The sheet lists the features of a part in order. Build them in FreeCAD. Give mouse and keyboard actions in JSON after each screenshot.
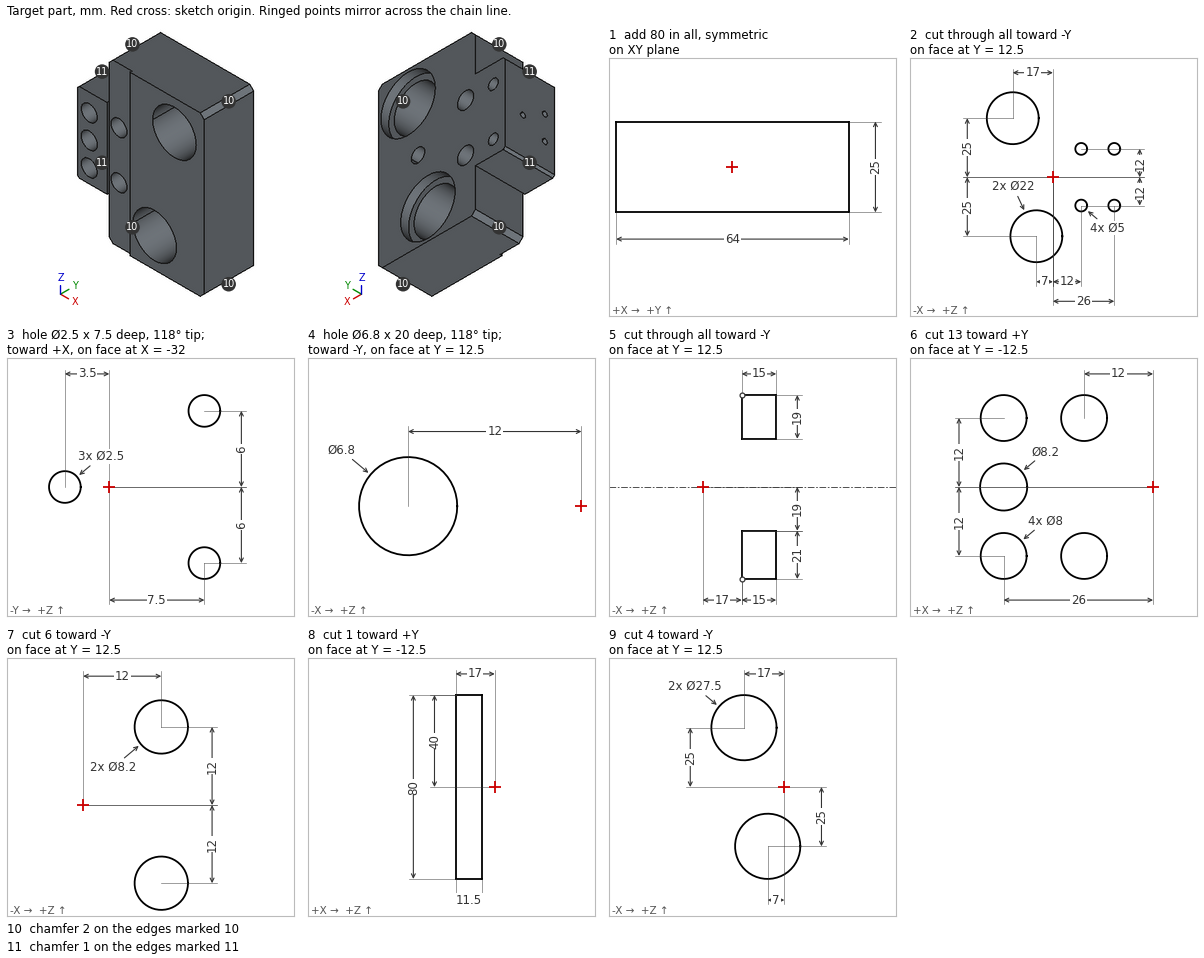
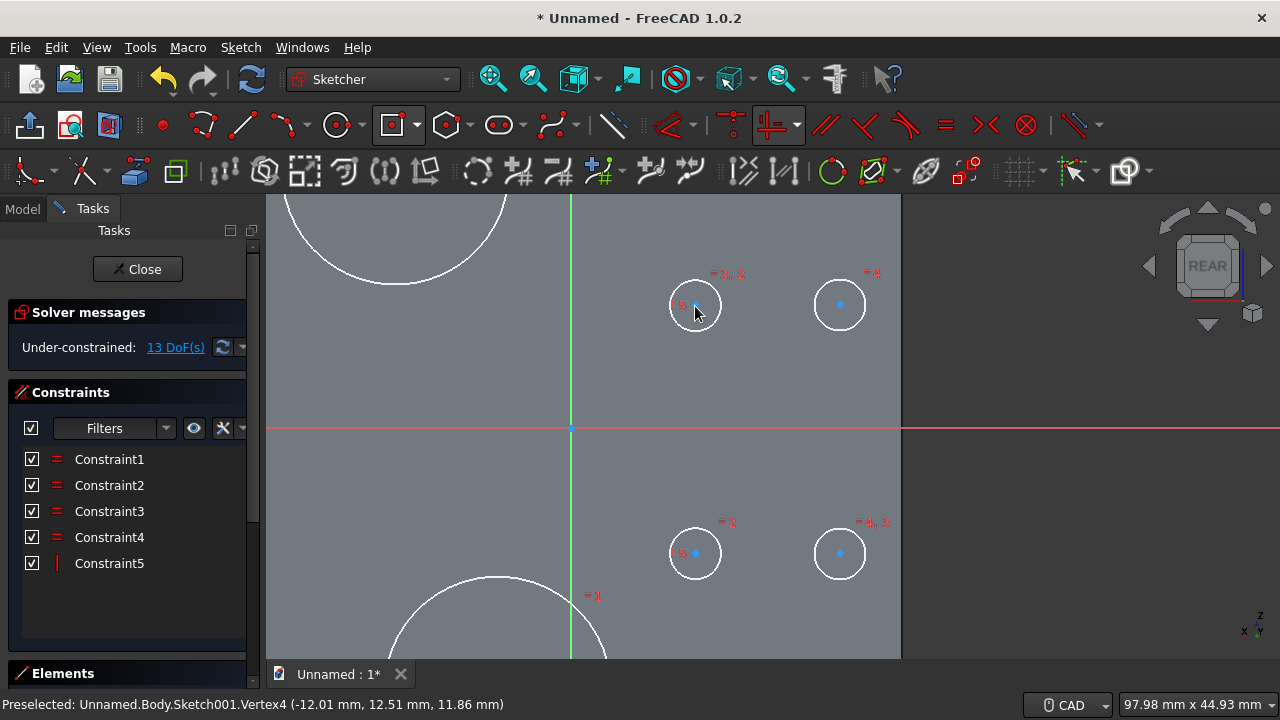
{"action": "left_click", "coordinate": [695, 554]}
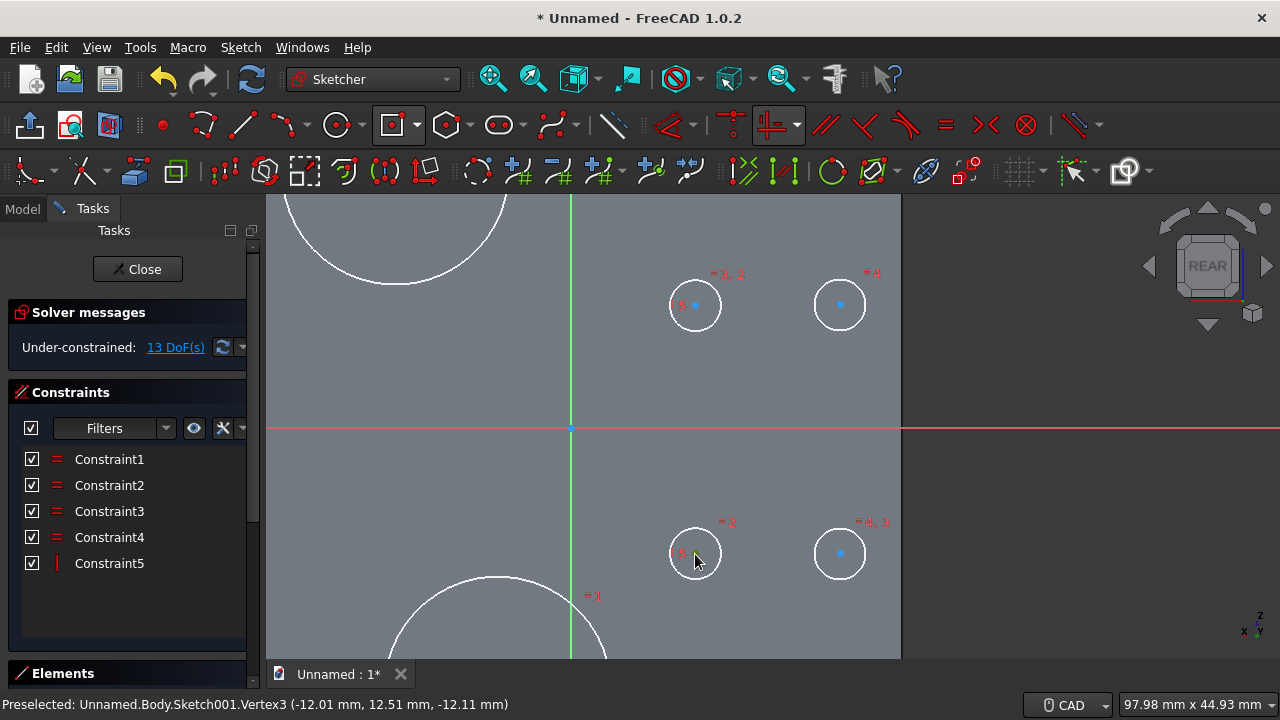
{"action": "left_click", "coordinate": [840, 554]}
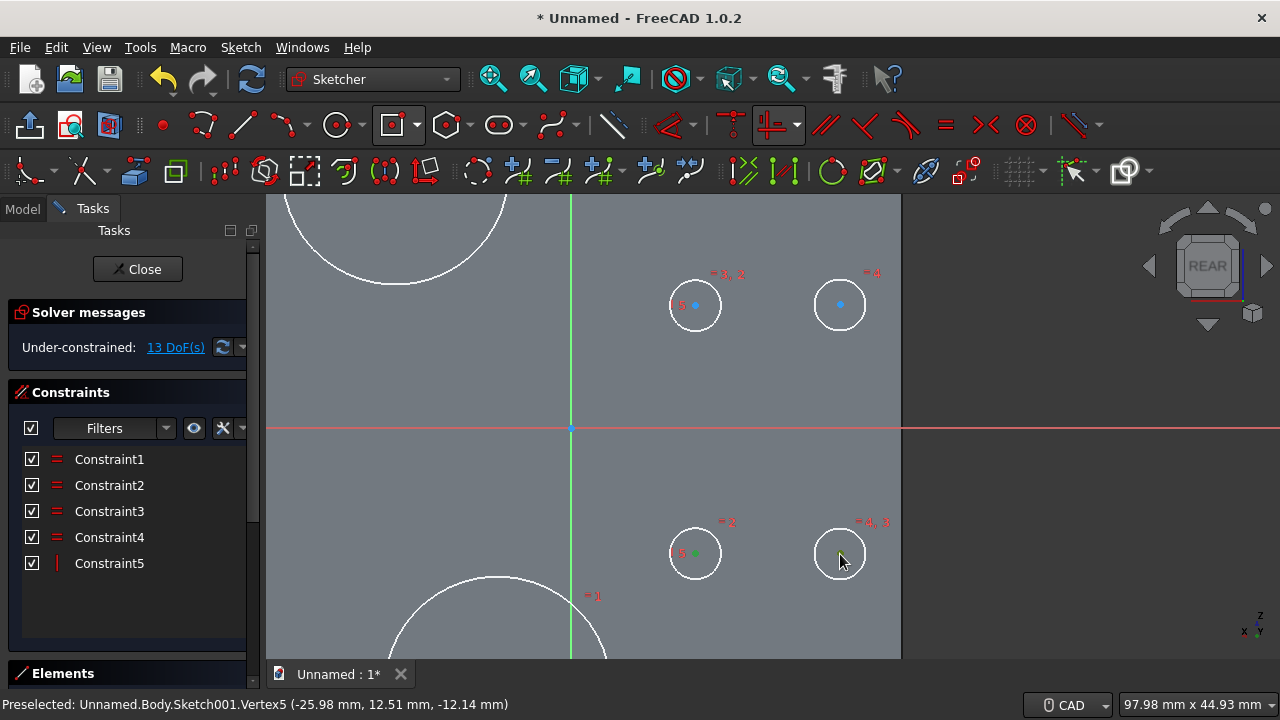
{"action": "key", "text": "h"}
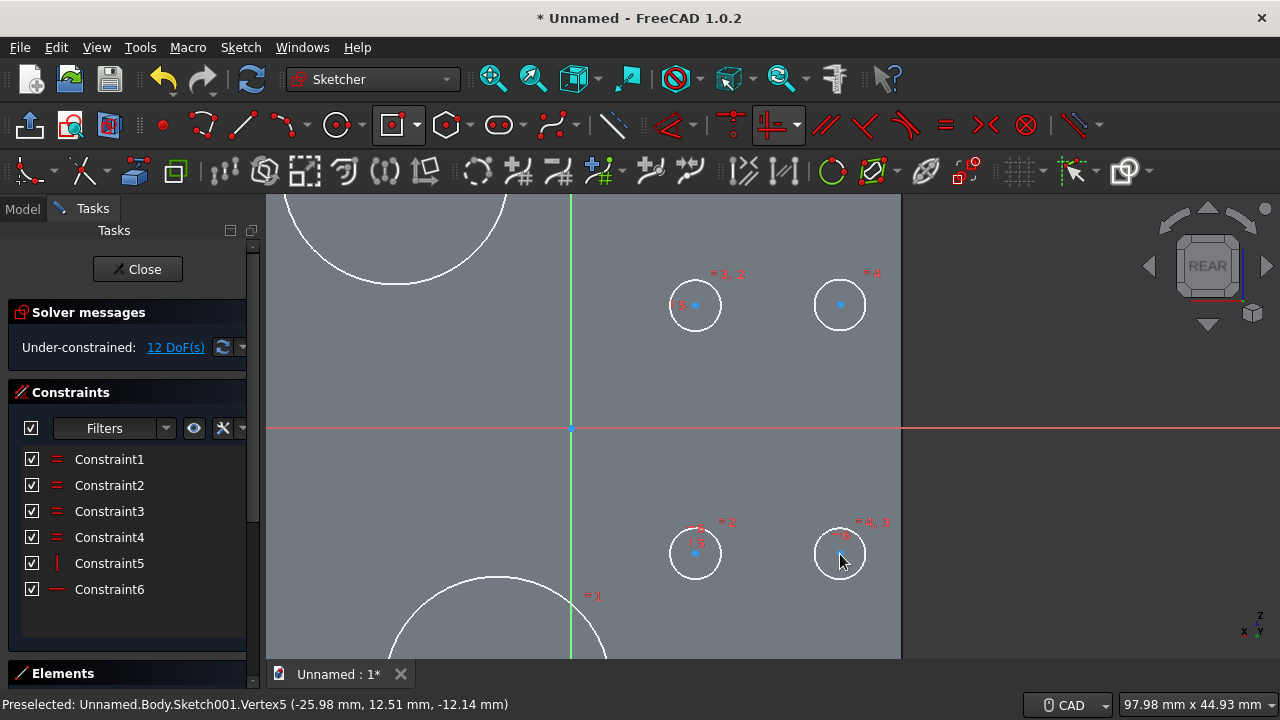
{"action": "left_click", "coordinate": [840, 554]}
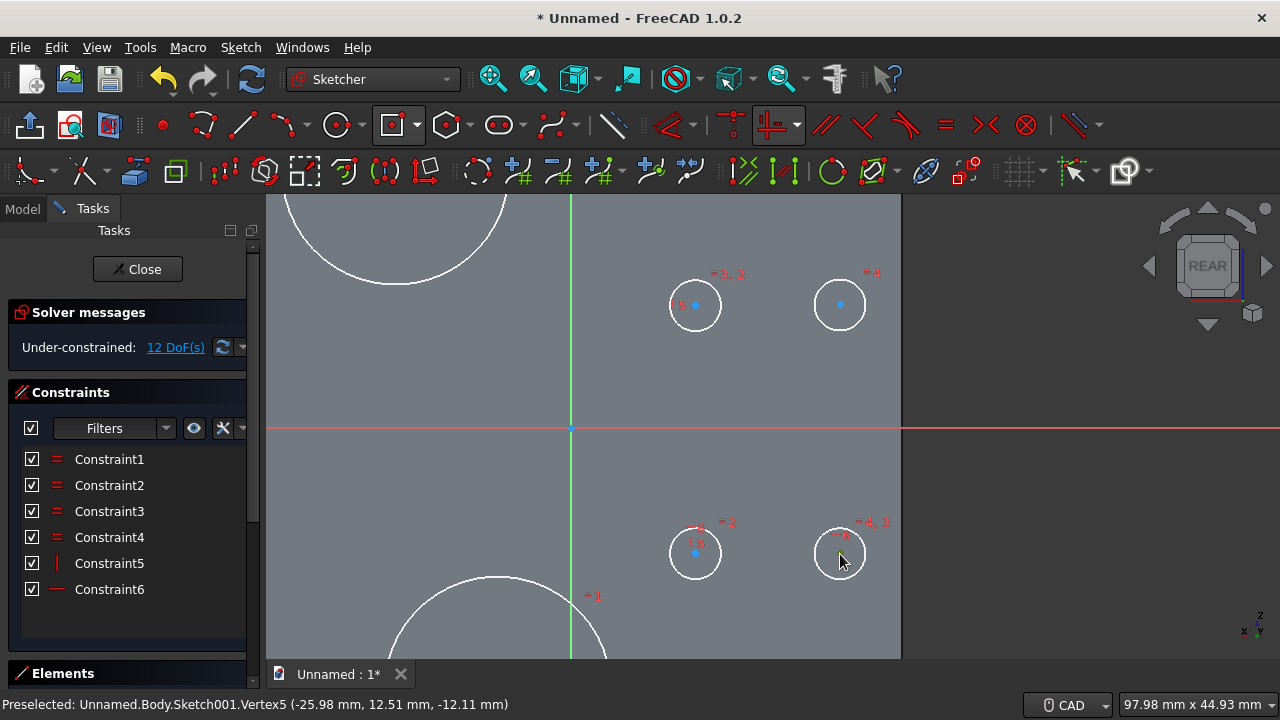
{"action": "left_click", "coordinate": [840, 305]}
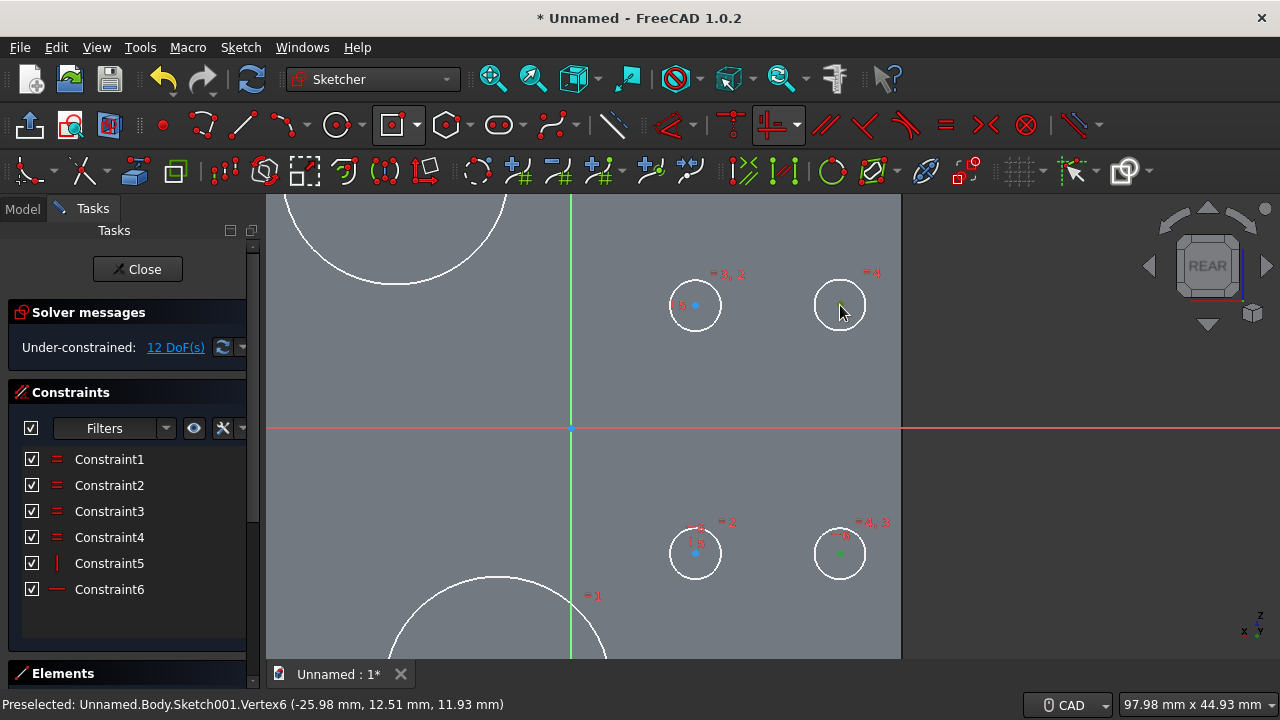
{"action": "left_click", "coordinate": [800, 126]}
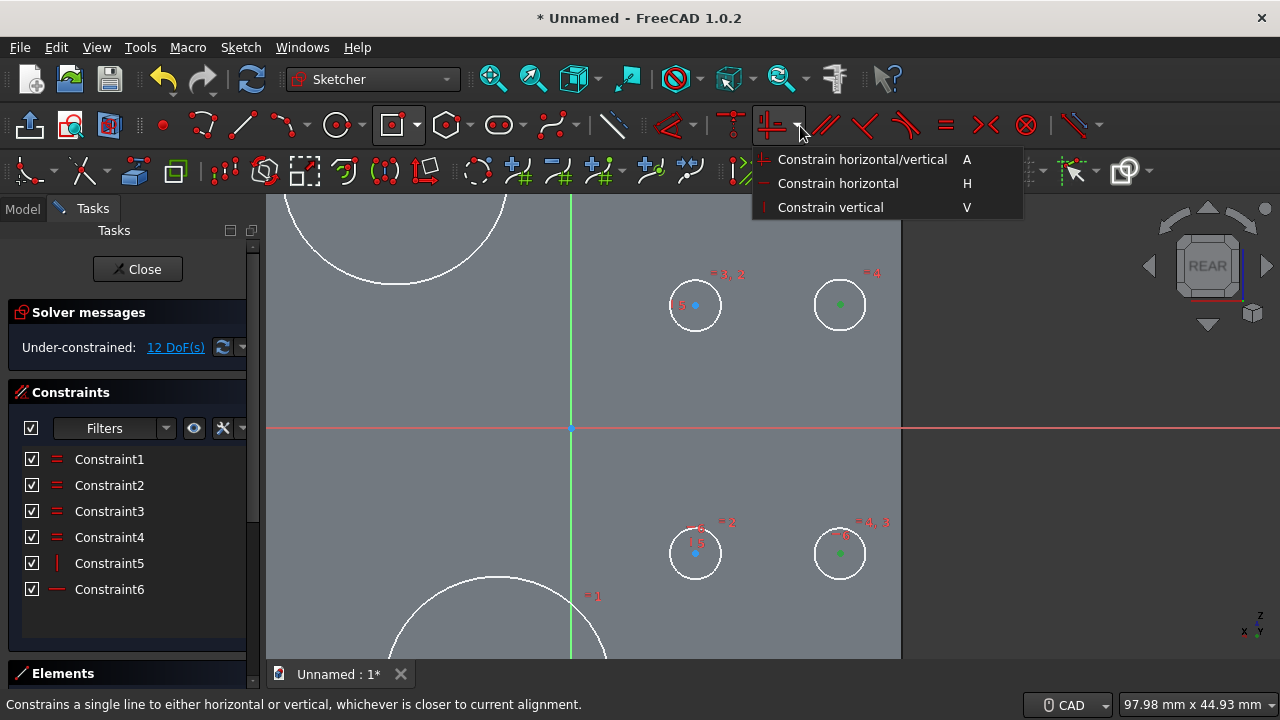
{"action": "left_click", "coordinate": [888, 207]}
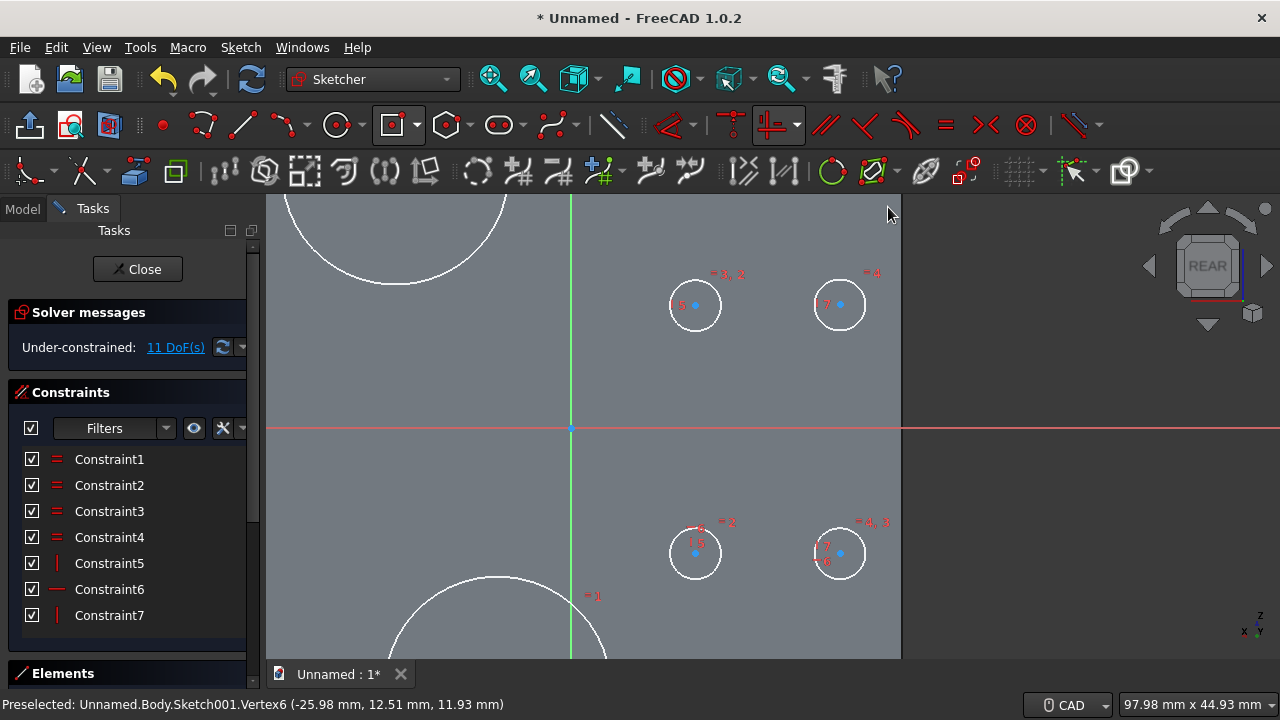
{"action": "left_click", "coordinate": [695, 306]}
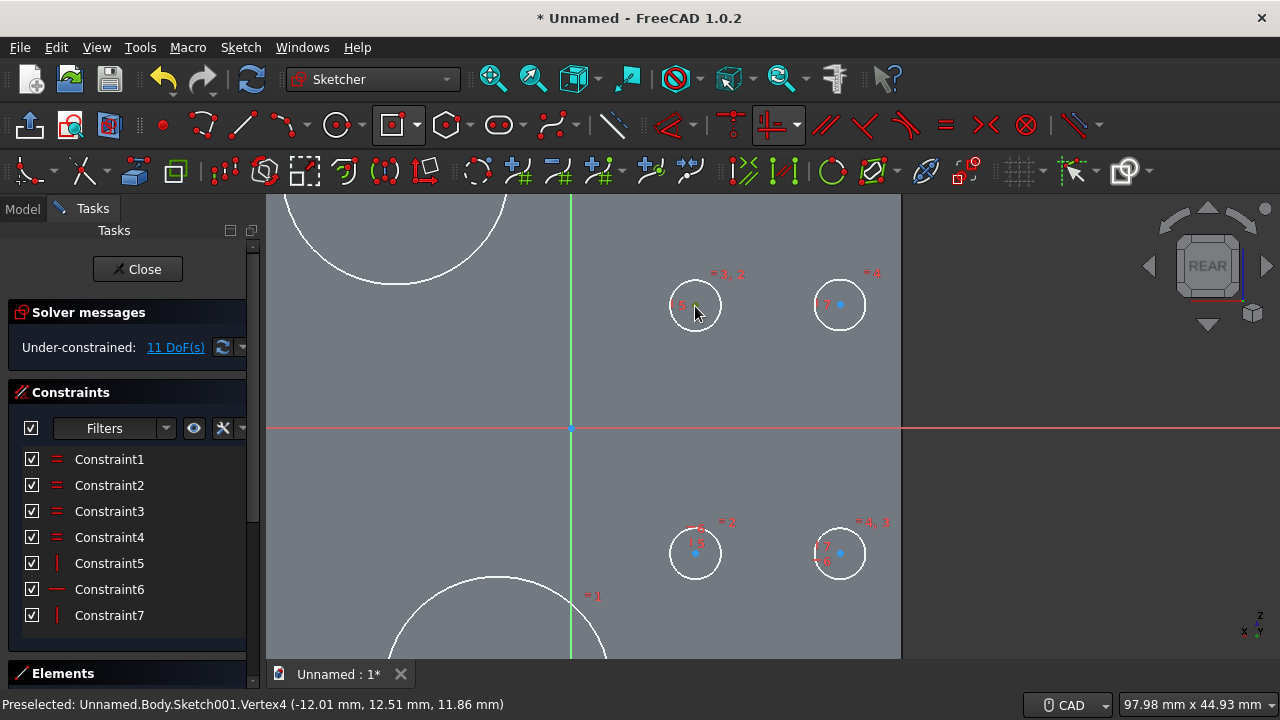
{"action": "left_click", "coordinate": [840, 305]}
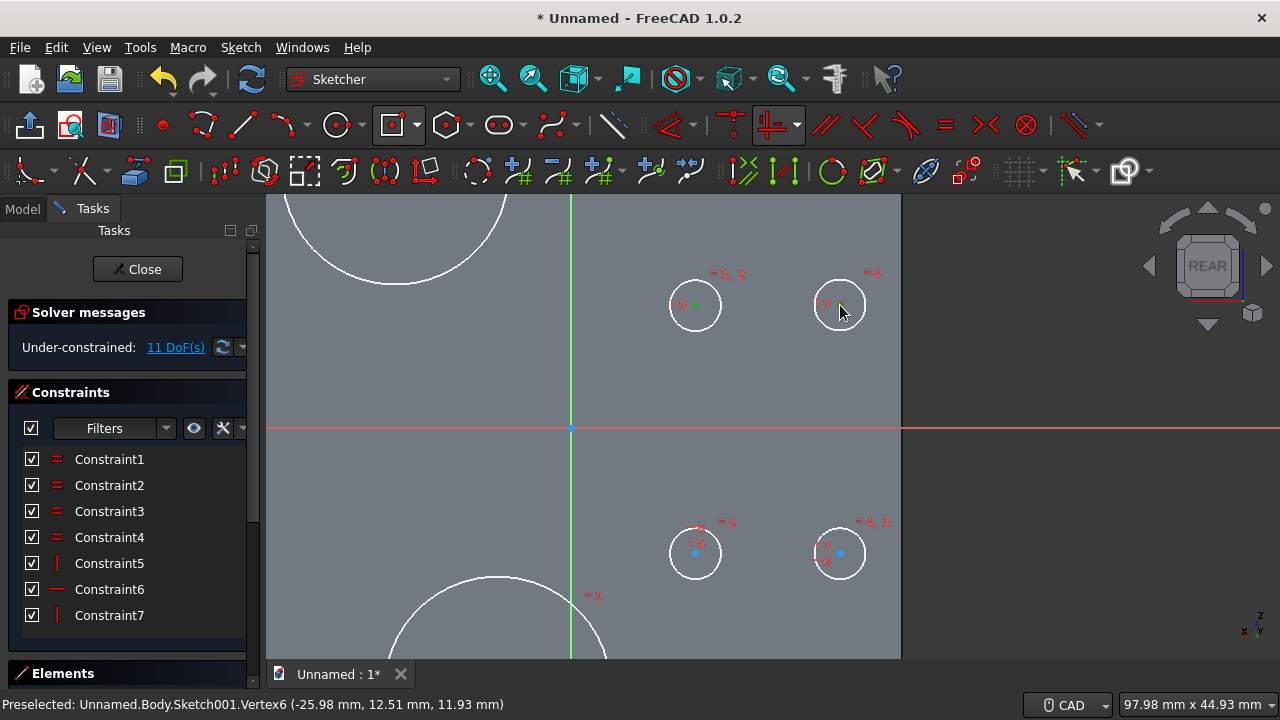
{"action": "left_click", "coordinate": [800, 126]}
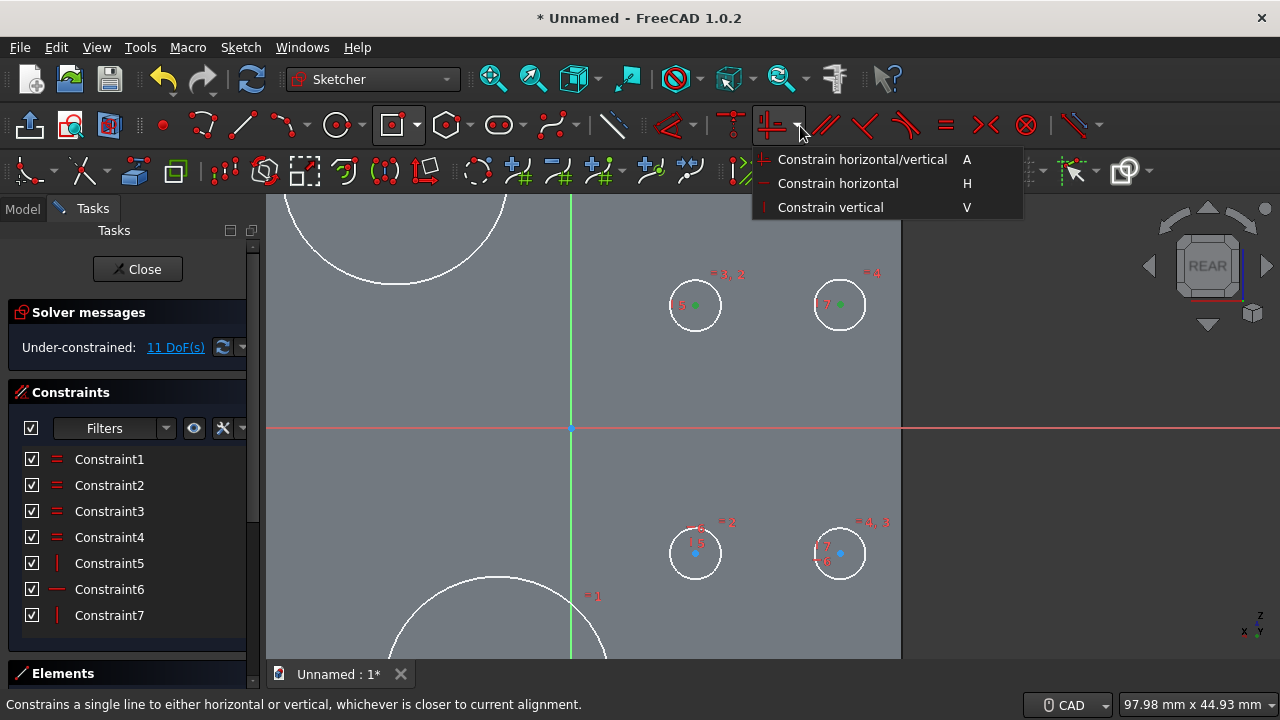
{"action": "left_click", "coordinate": [888, 183]}